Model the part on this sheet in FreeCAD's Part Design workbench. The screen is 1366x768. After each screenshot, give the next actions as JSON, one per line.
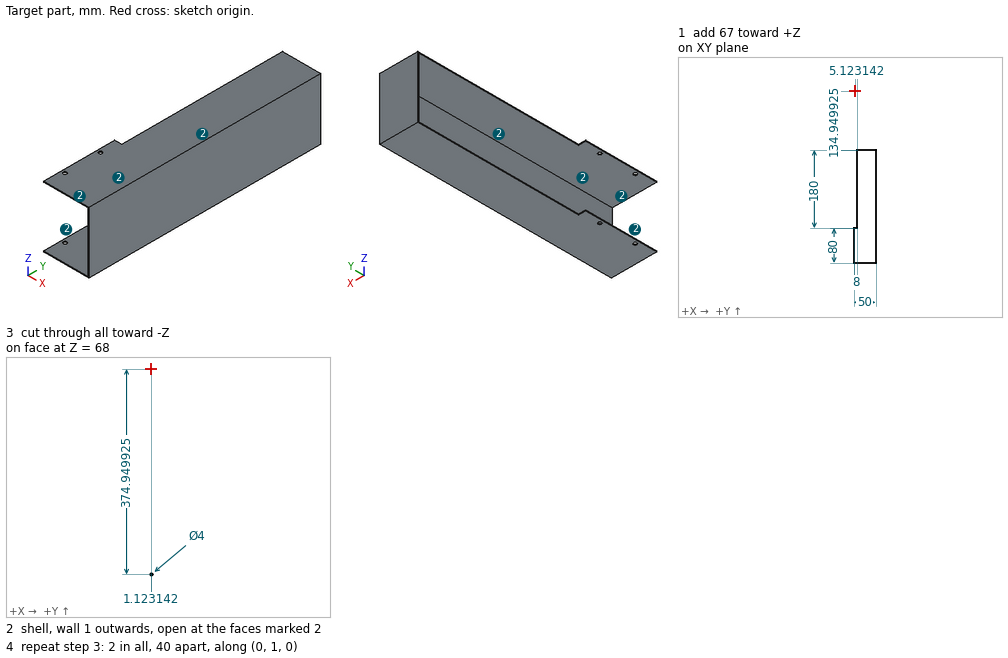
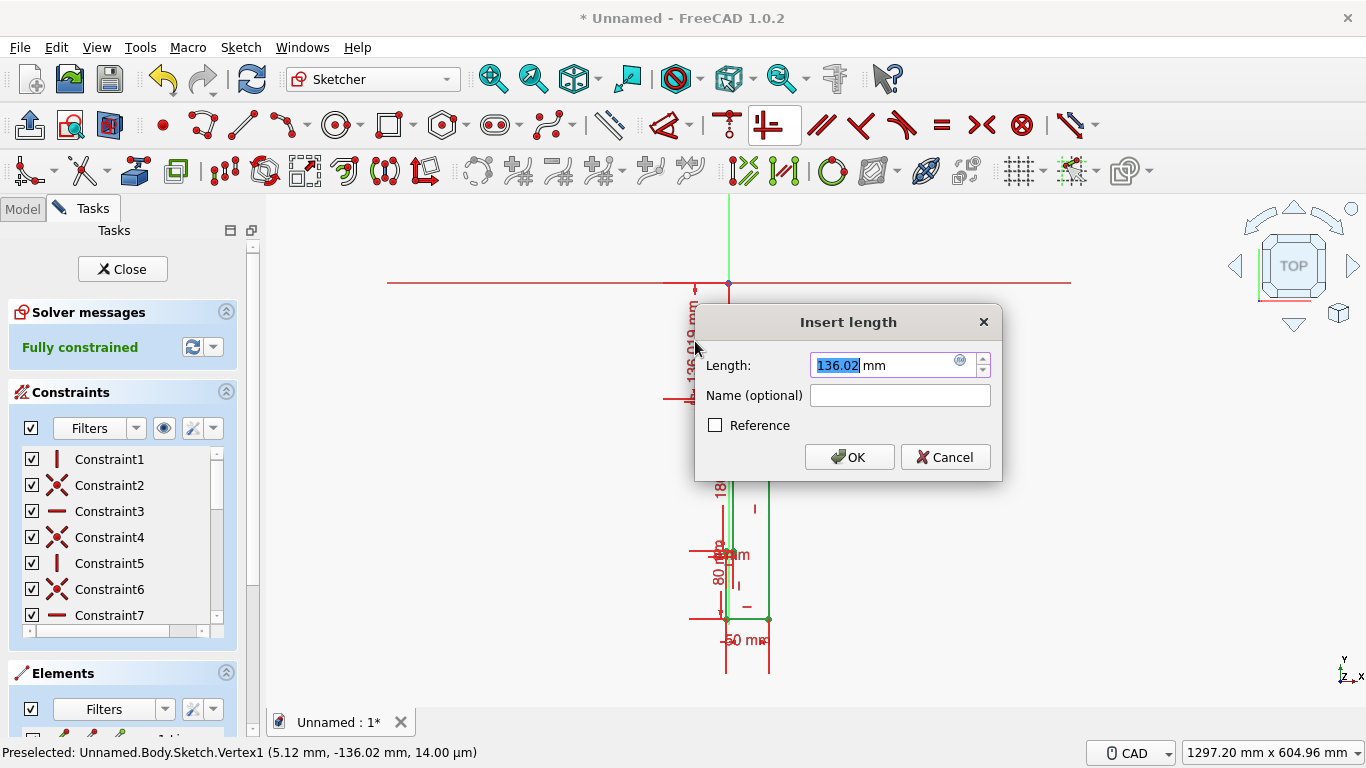
{"action": "type", "text": "134.949925"}
{"action": "key", "text": "Return"}
{"action": "key", "text": "Escape"}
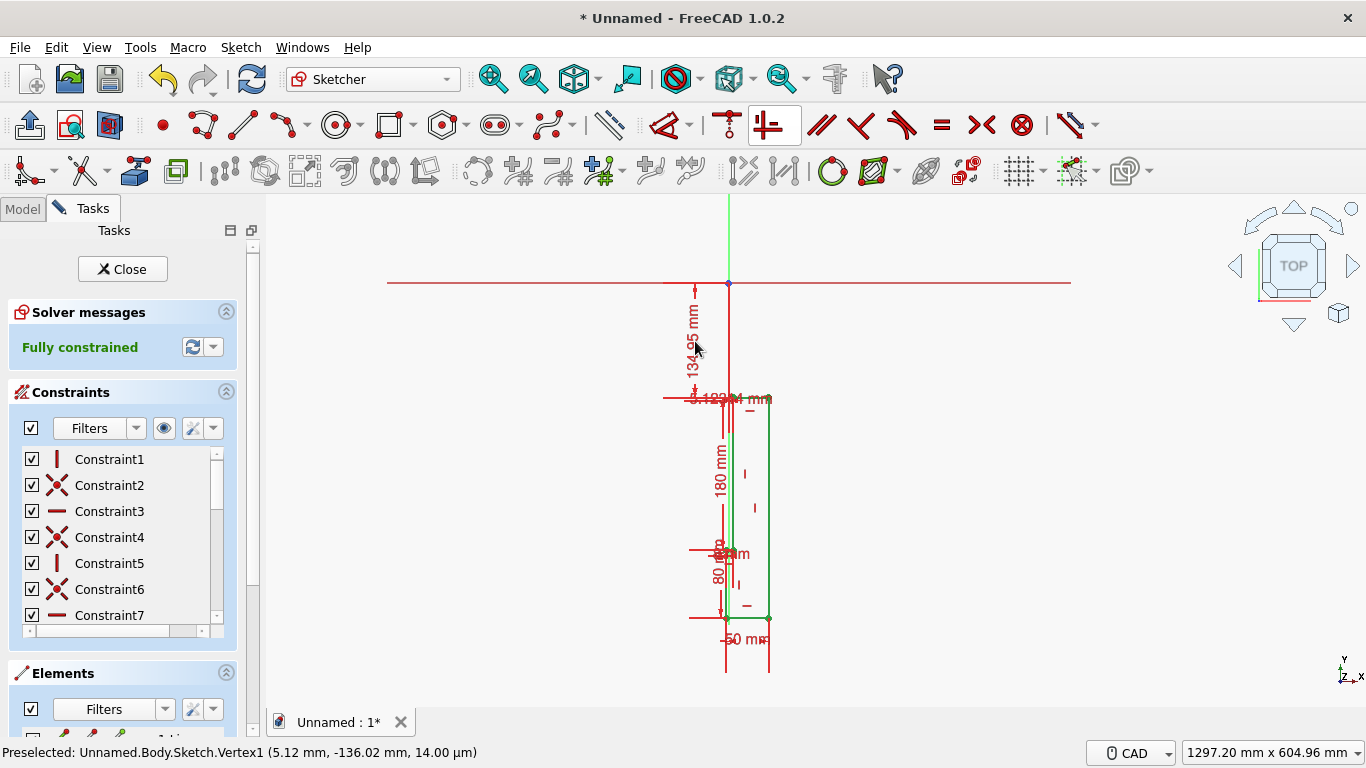
{"action": "left_click", "coordinate": [123, 269]}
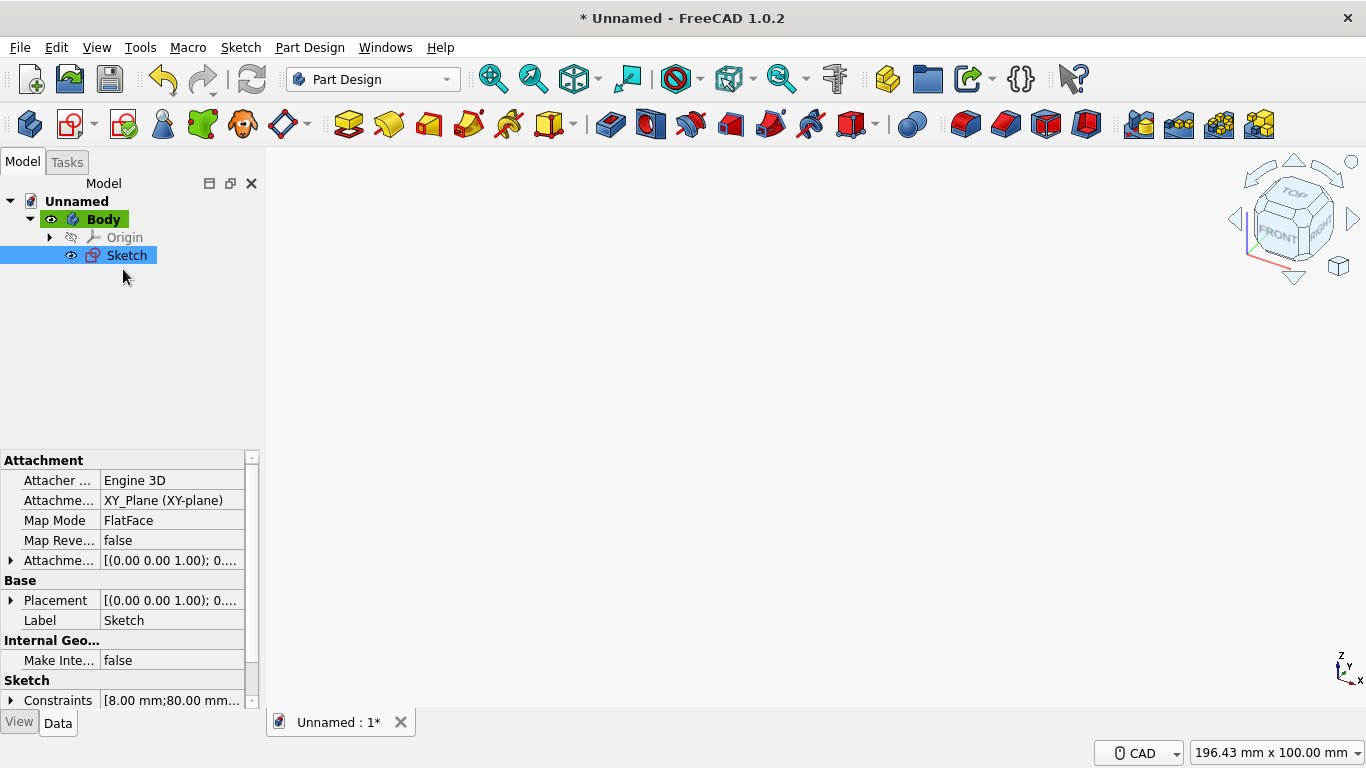
{"action": "left_click", "coordinate": [350, 124]}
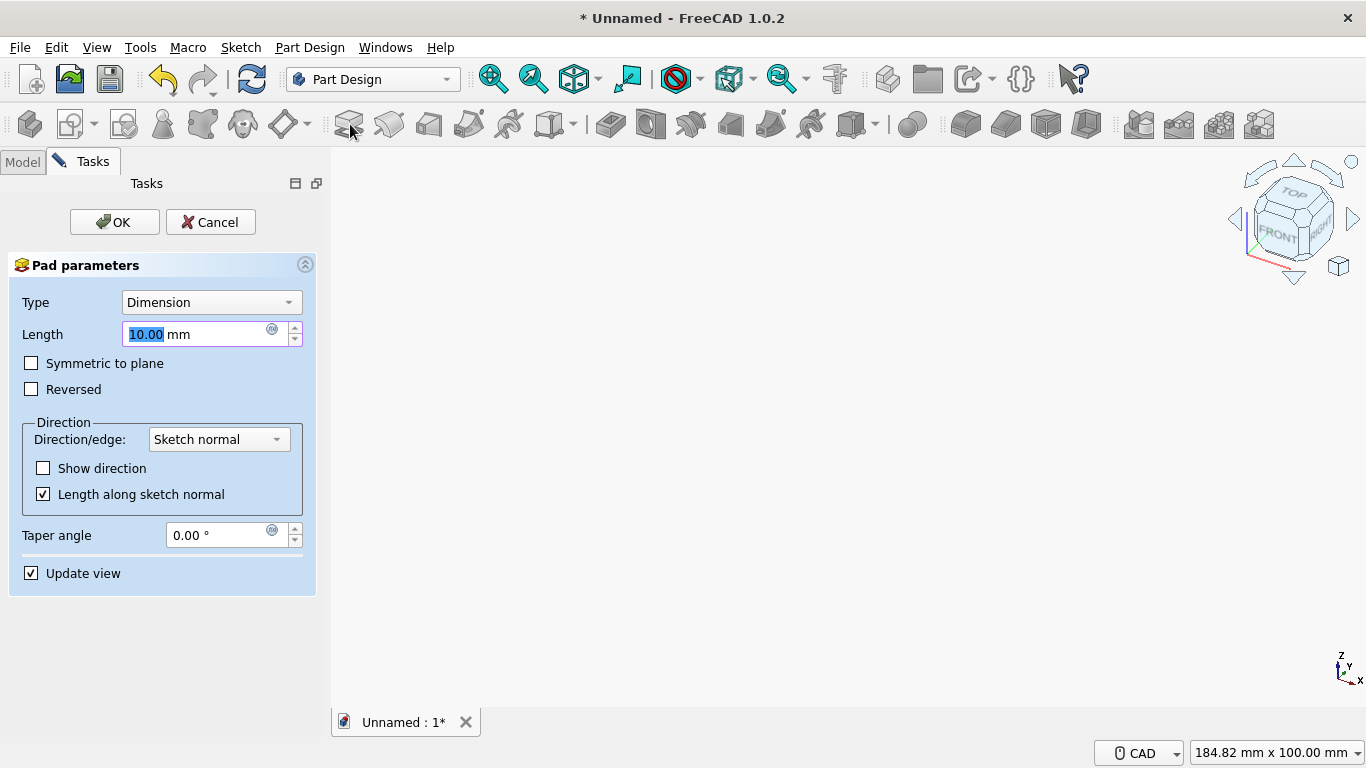
{"action": "type", "text": "67"}
{"action": "key", "text": "Tab"}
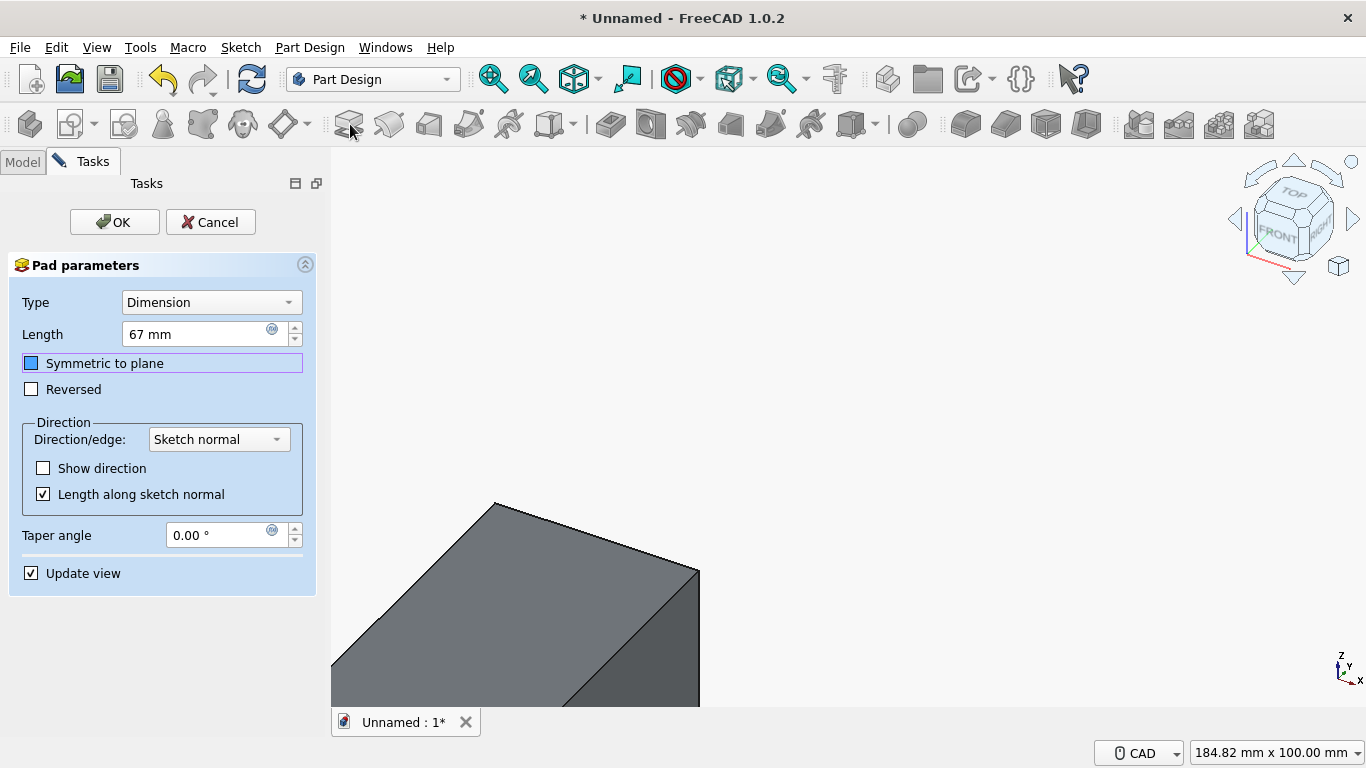
{"action": "left_click", "coordinate": [115, 222]}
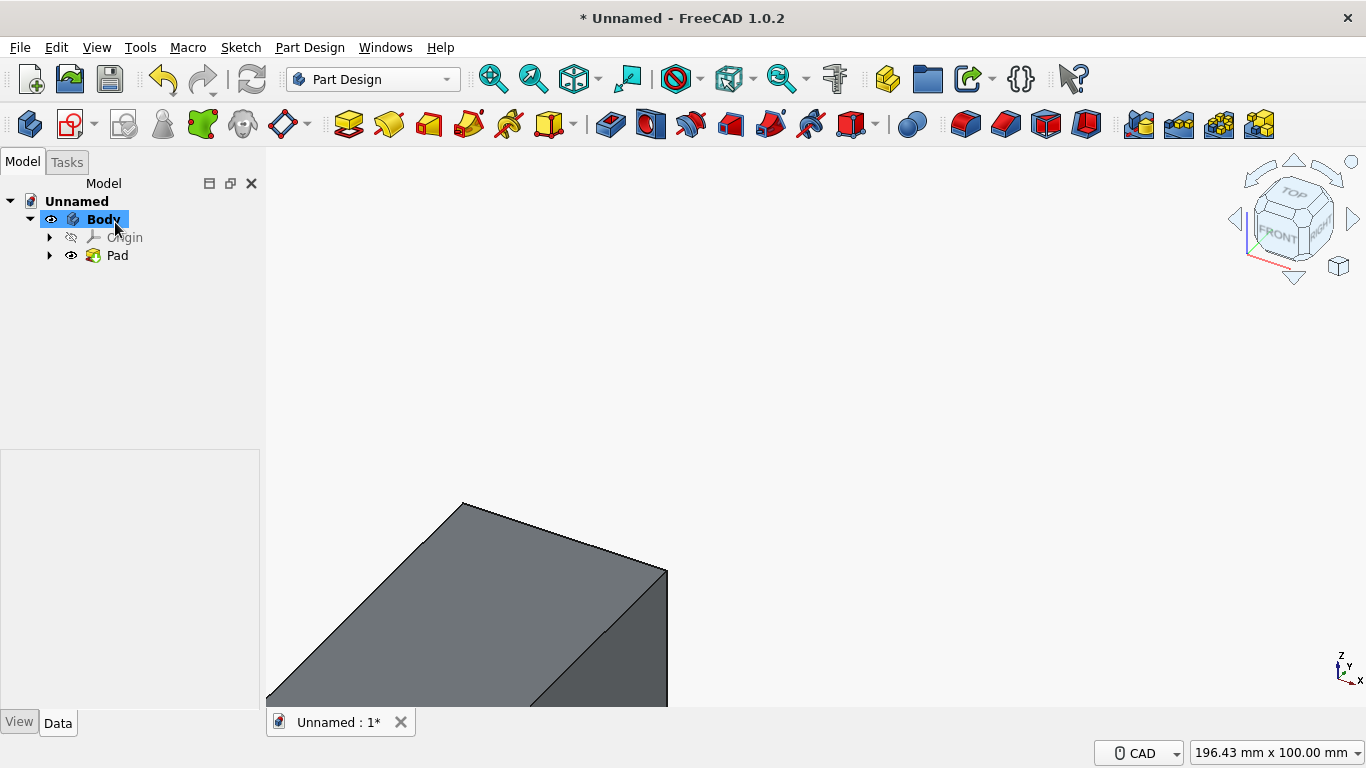
{"action": "left_click", "coordinate": [494, 80]}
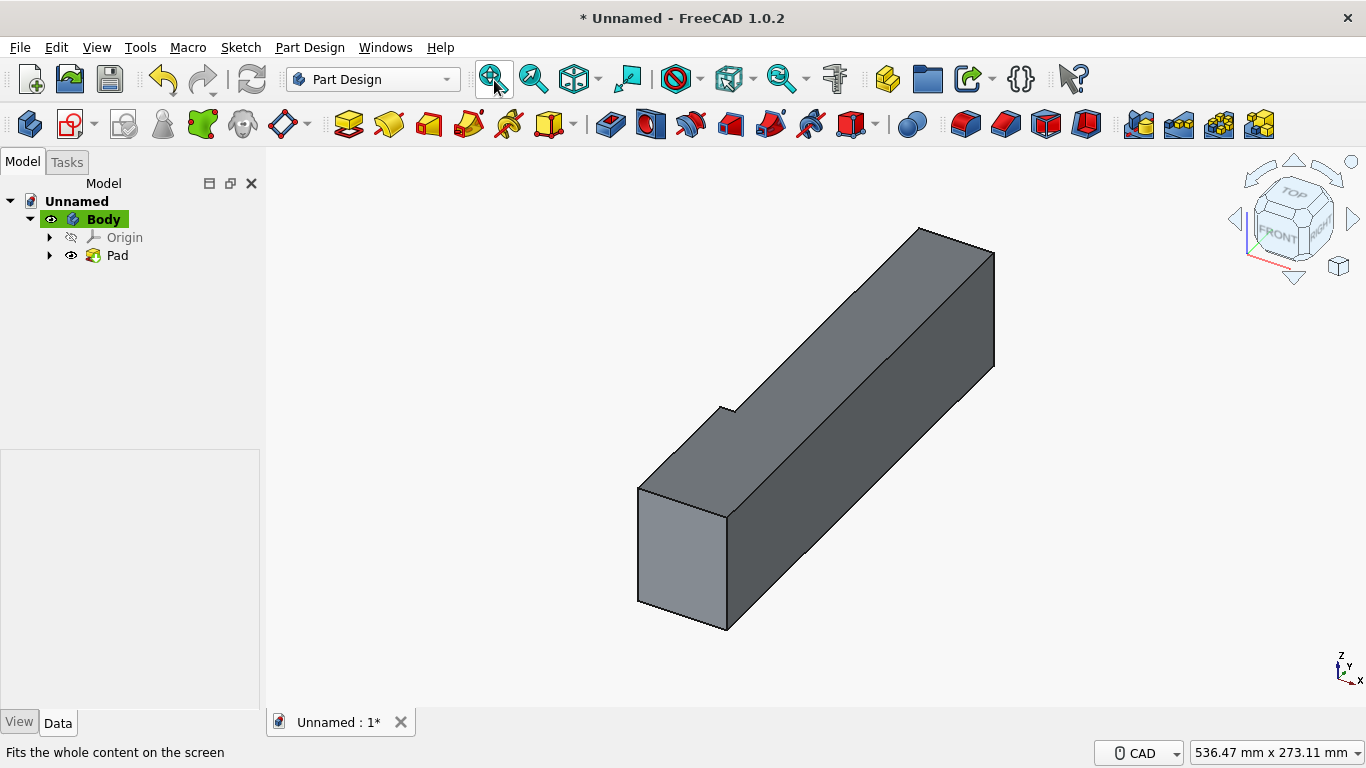
{"action": "left_click", "coordinate": [683, 558]}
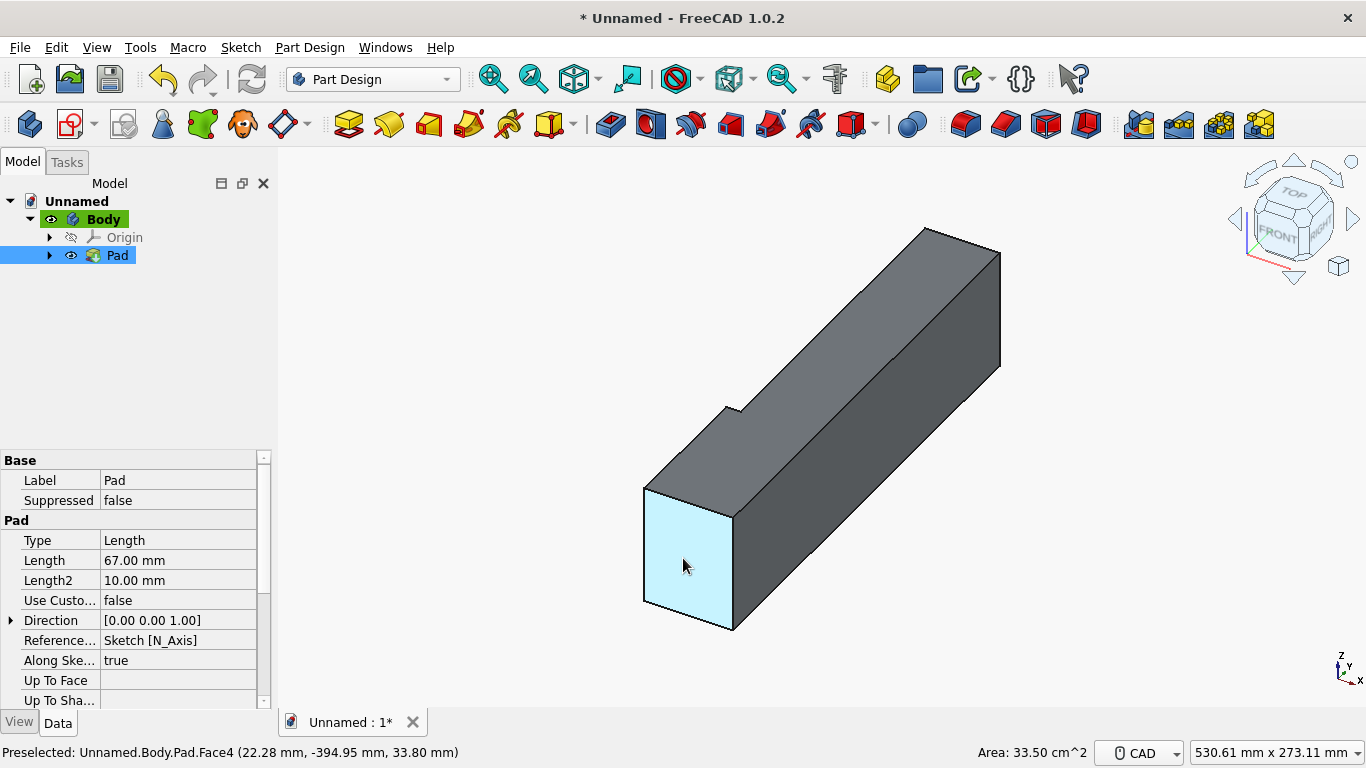
{"action": "key", "text": "0"}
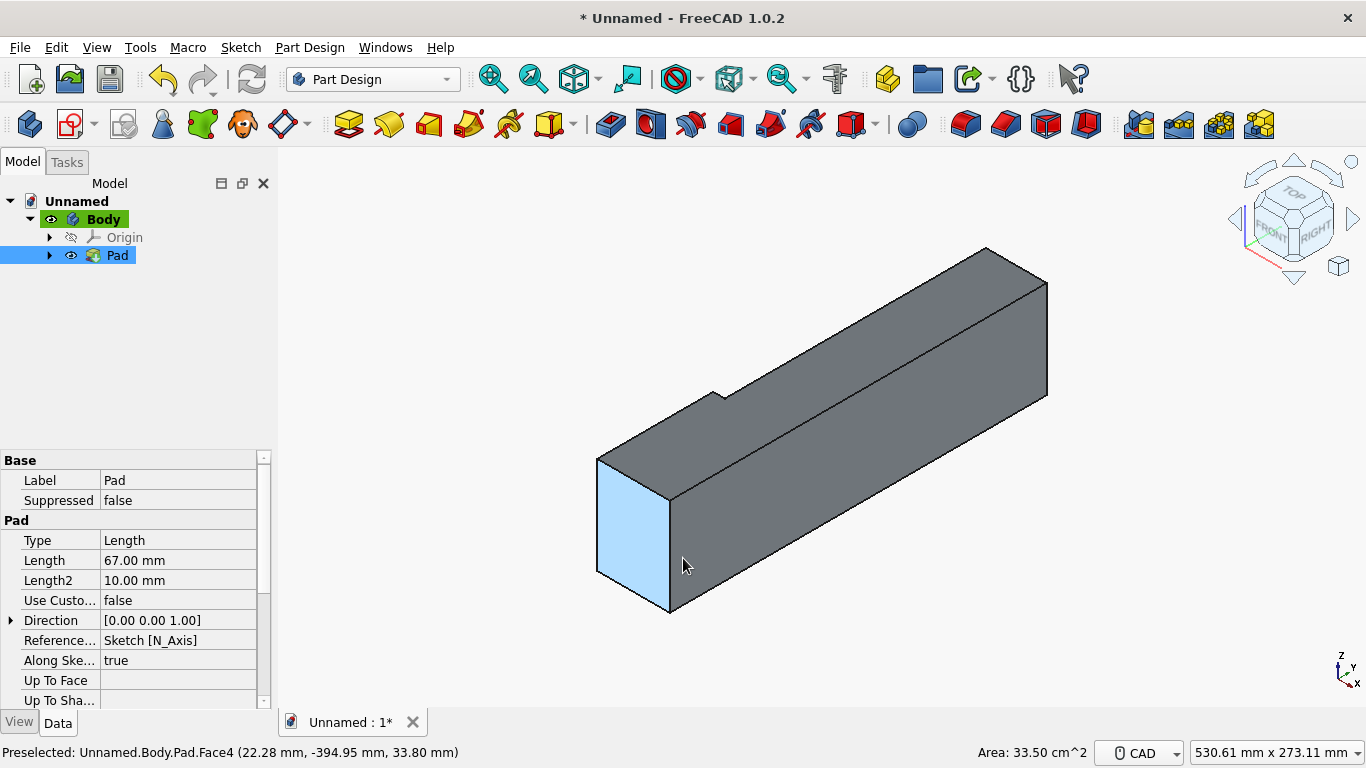
{"action": "key", "text": "2"}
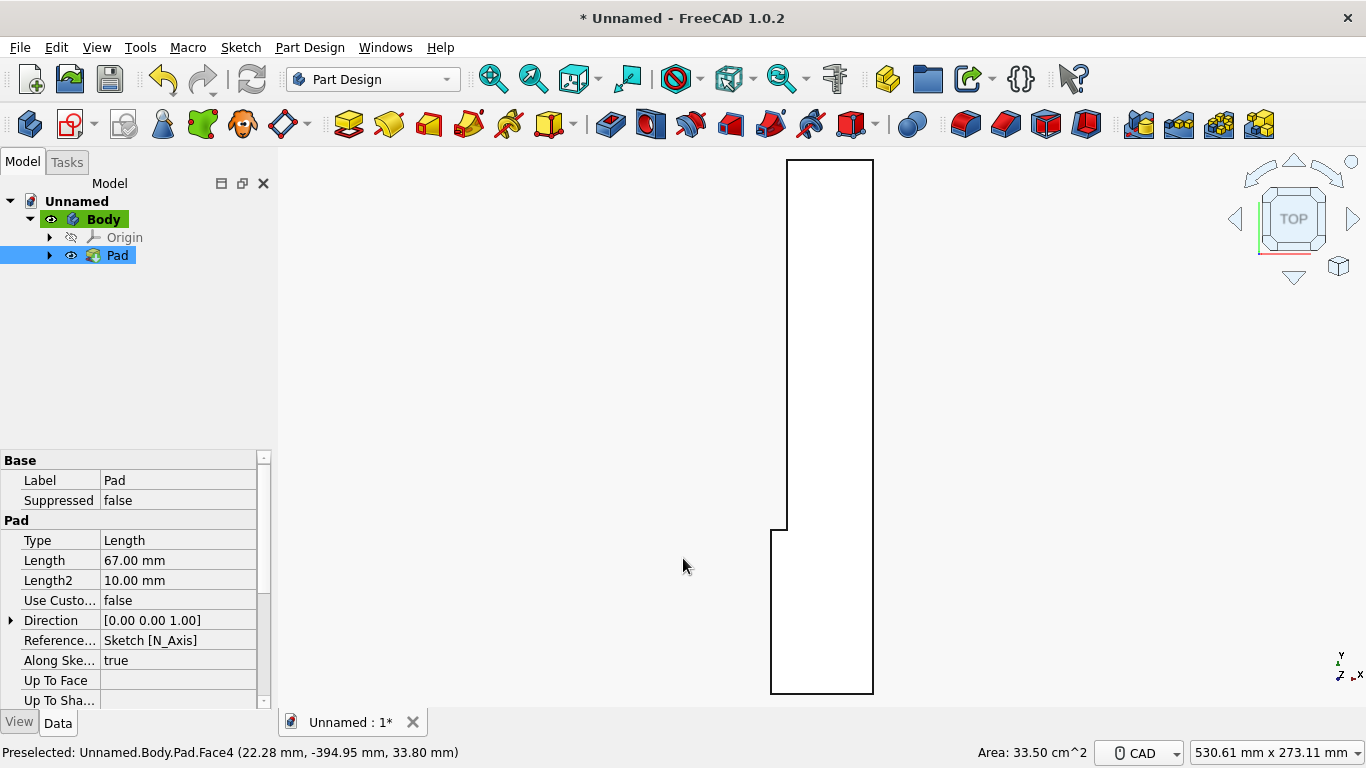
{"action": "key", "text": "1"}